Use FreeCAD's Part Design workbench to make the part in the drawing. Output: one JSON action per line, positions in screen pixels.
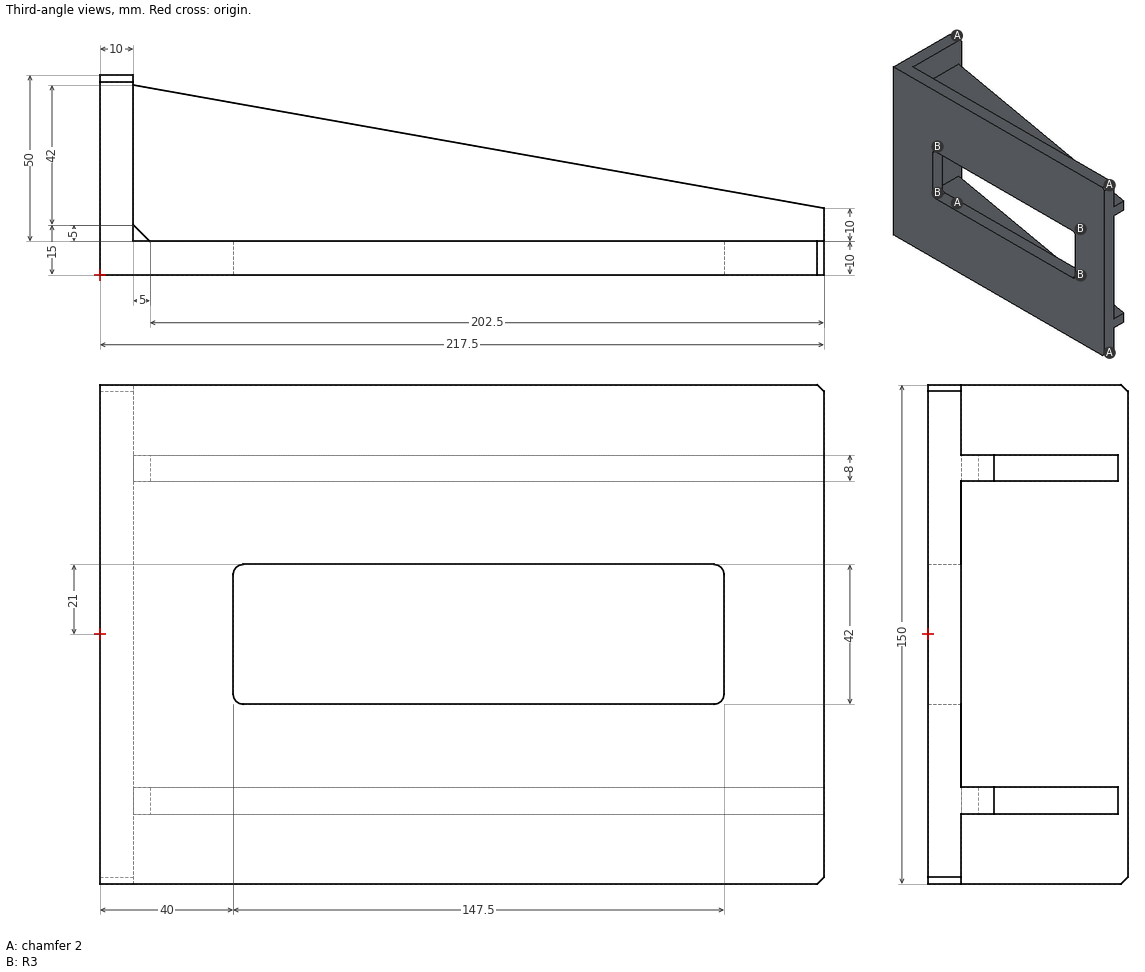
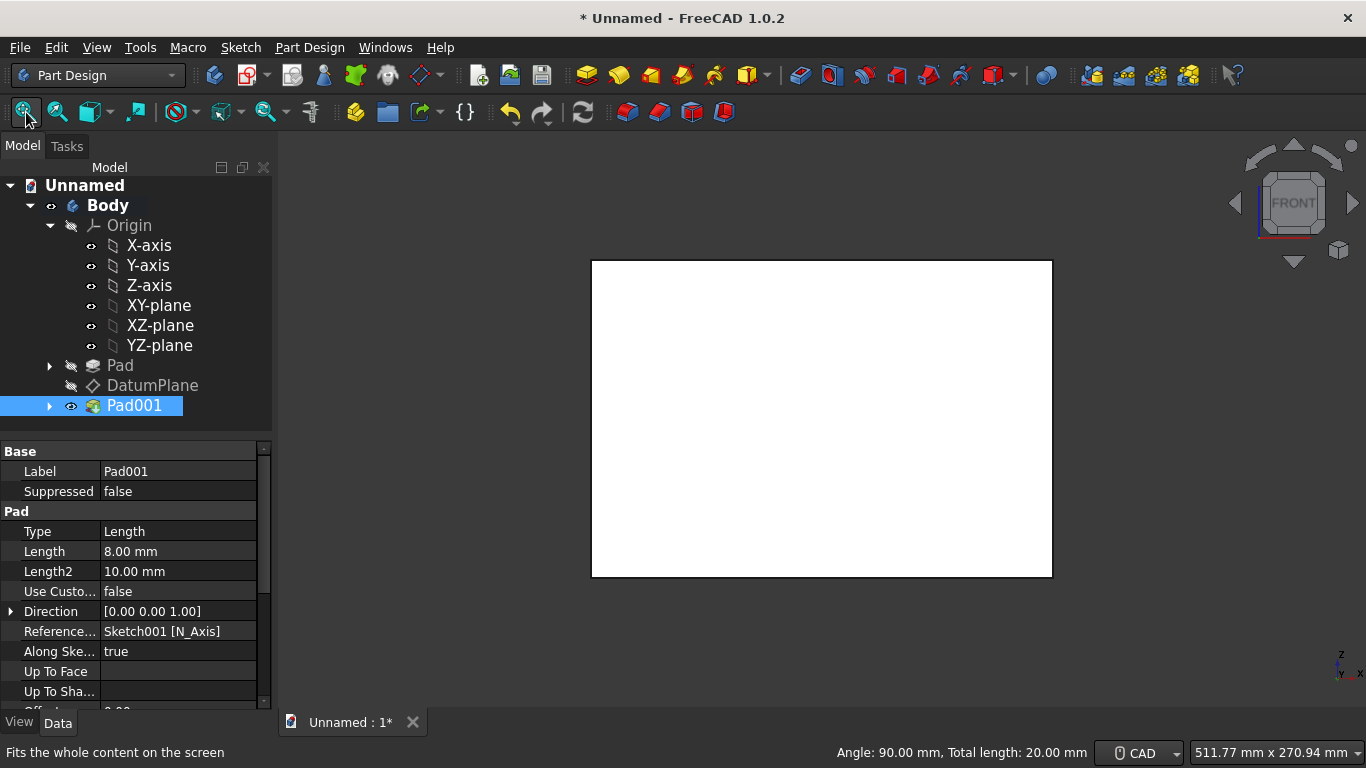
{"action": "scroll", "coordinate": [601, 577], "scroll_direction": "up", "scroll_amount": 4}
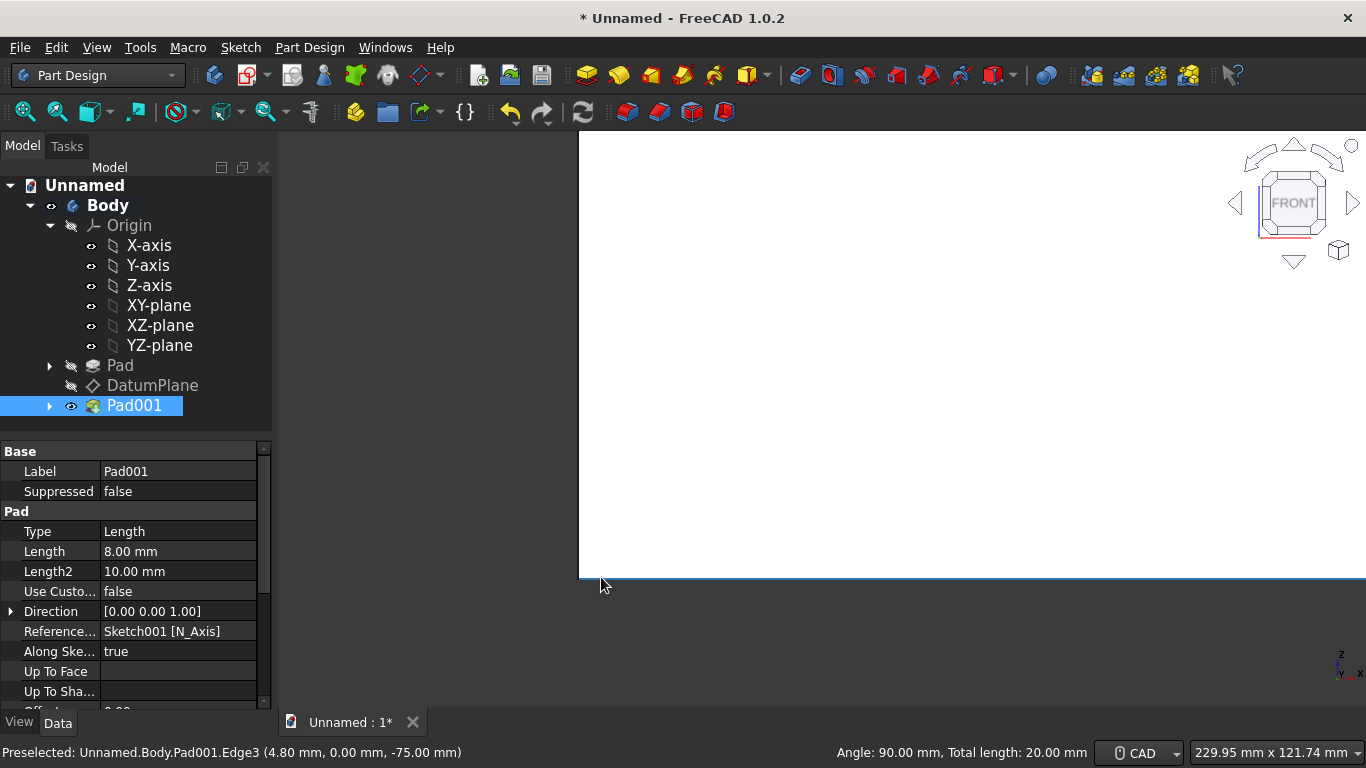
{"action": "left_click", "coordinate": [26, 112]}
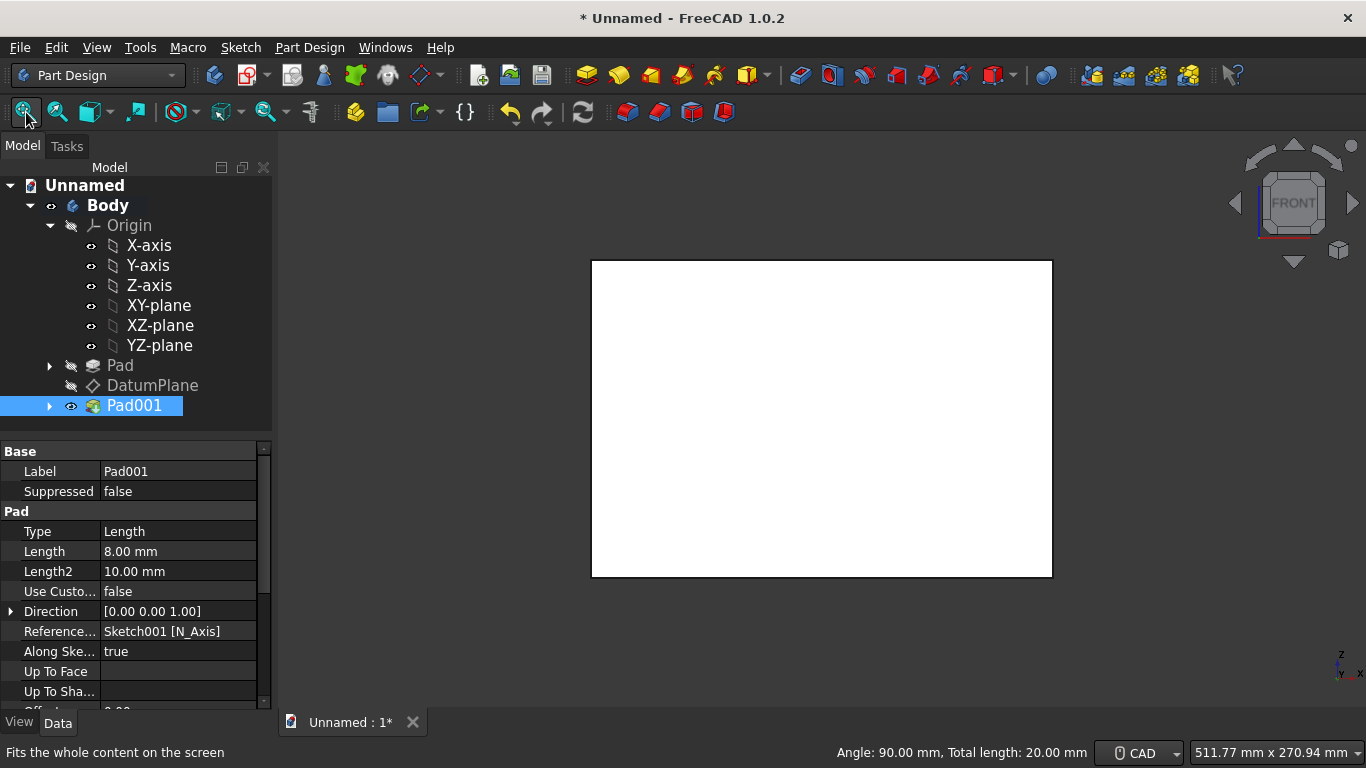
{"action": "key", "text": "3"}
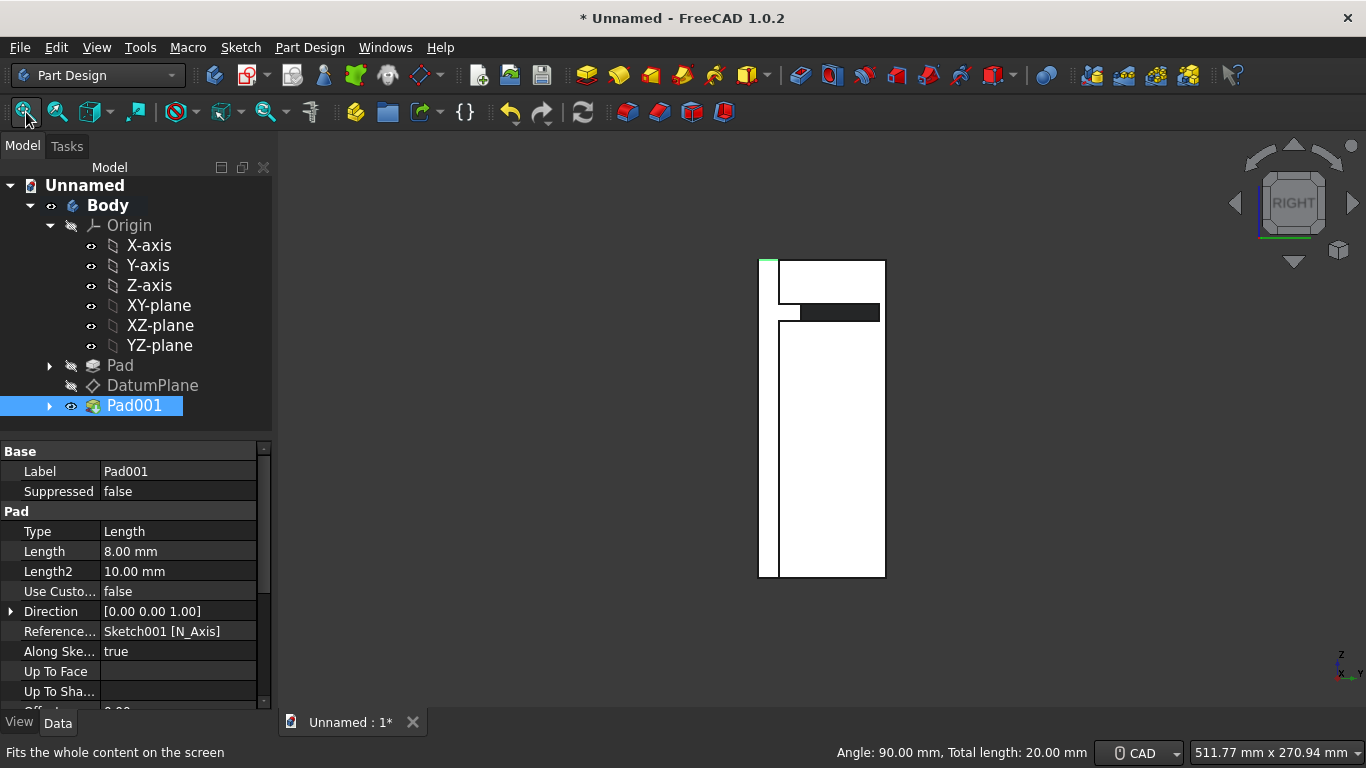
{"action": "left_click", "coordinate": [769, 577], "text": "ctrl"}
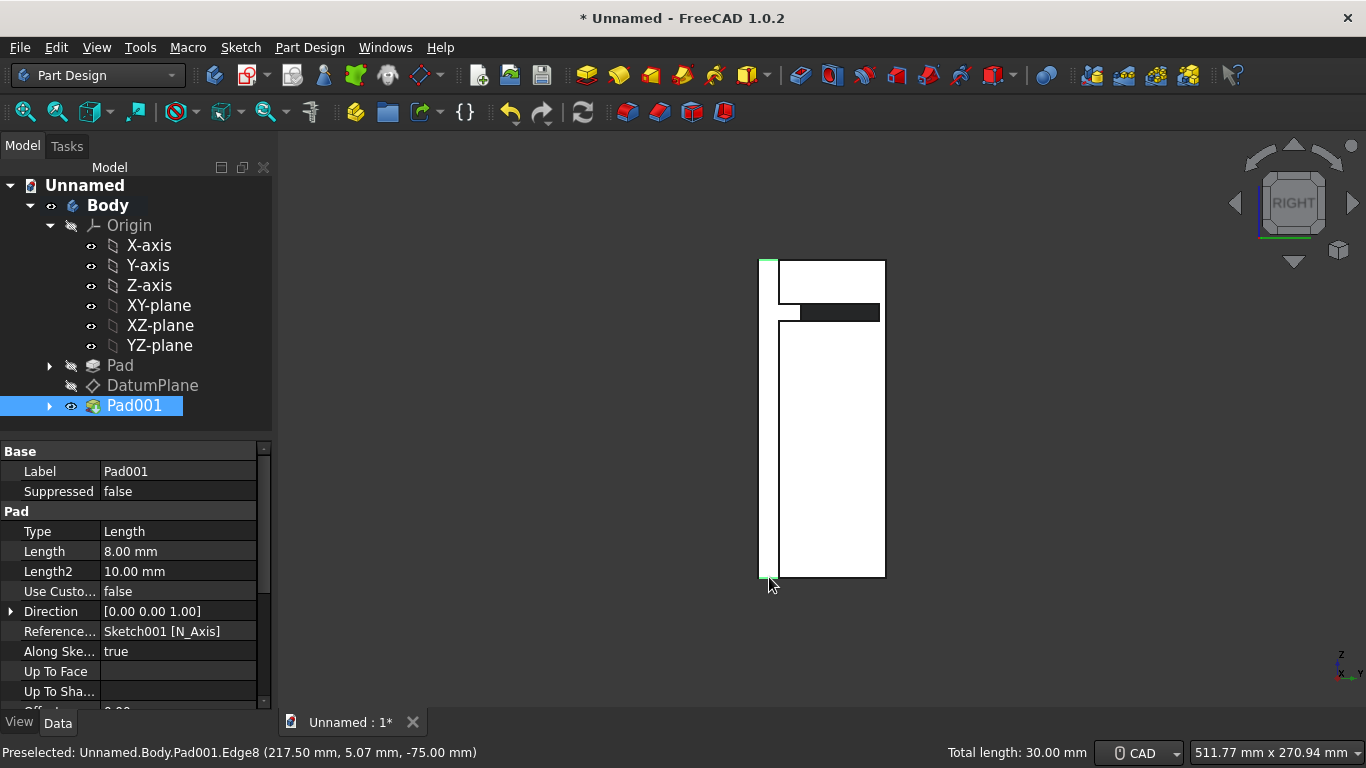
{"action": "scroll", "coordinate": [886, 577], "scroll_direction": "up", "scroll_amount": 4}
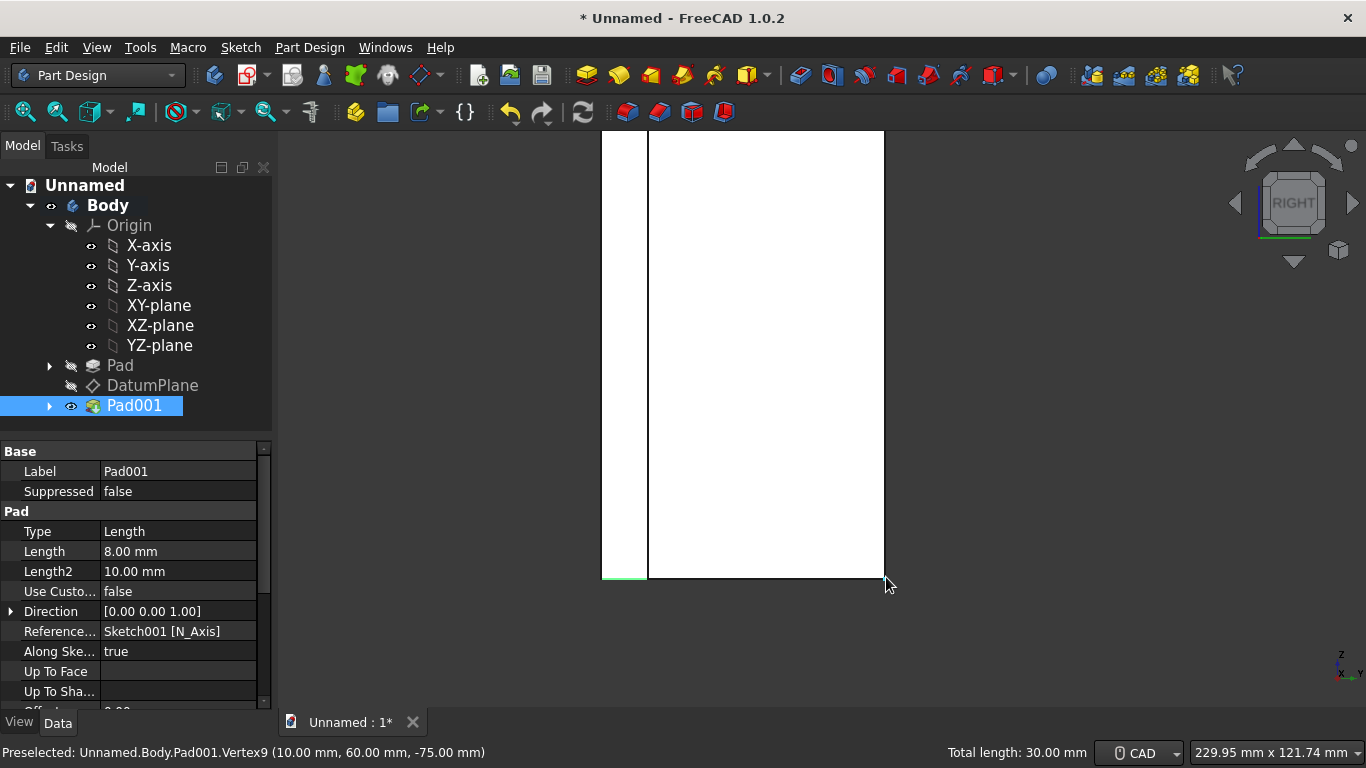
{"action": "left_click", "coordinate": [26, 112]}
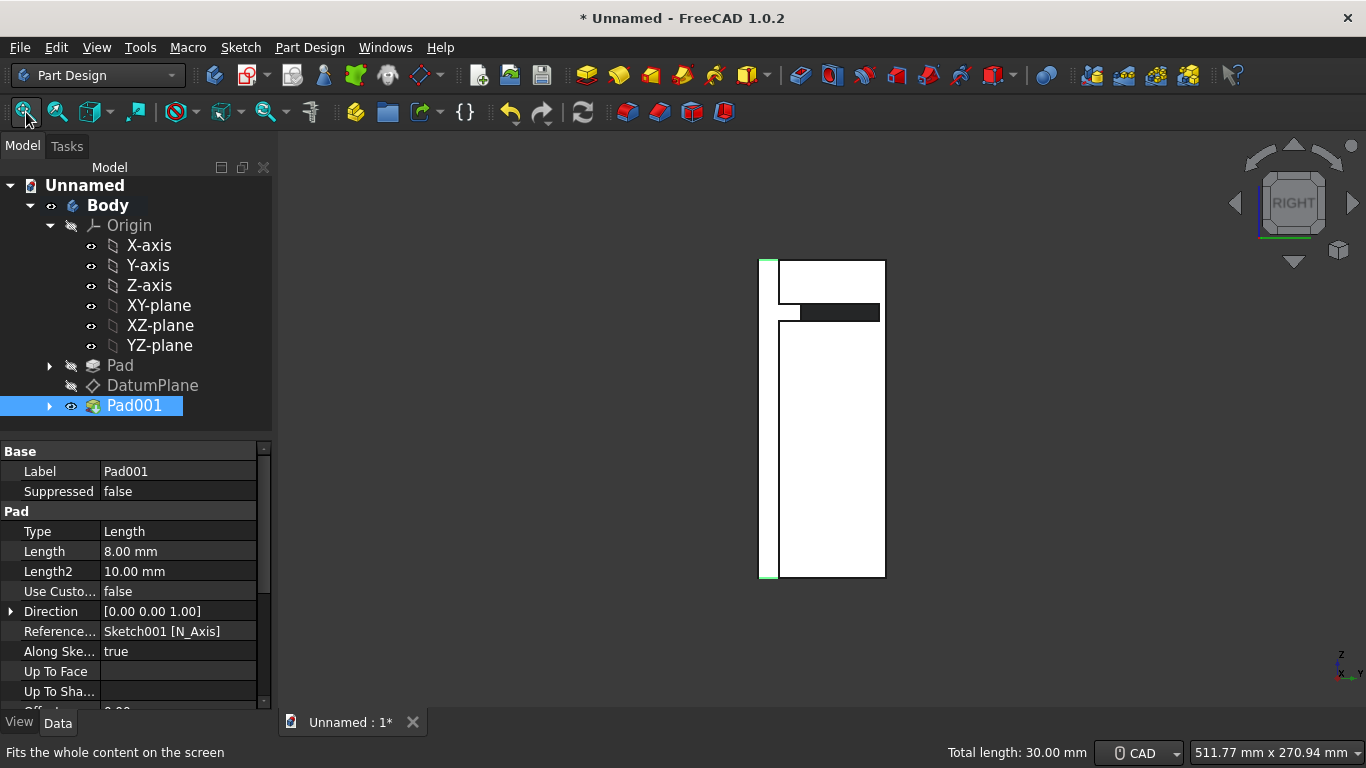
{"action": "key", "text": "5"}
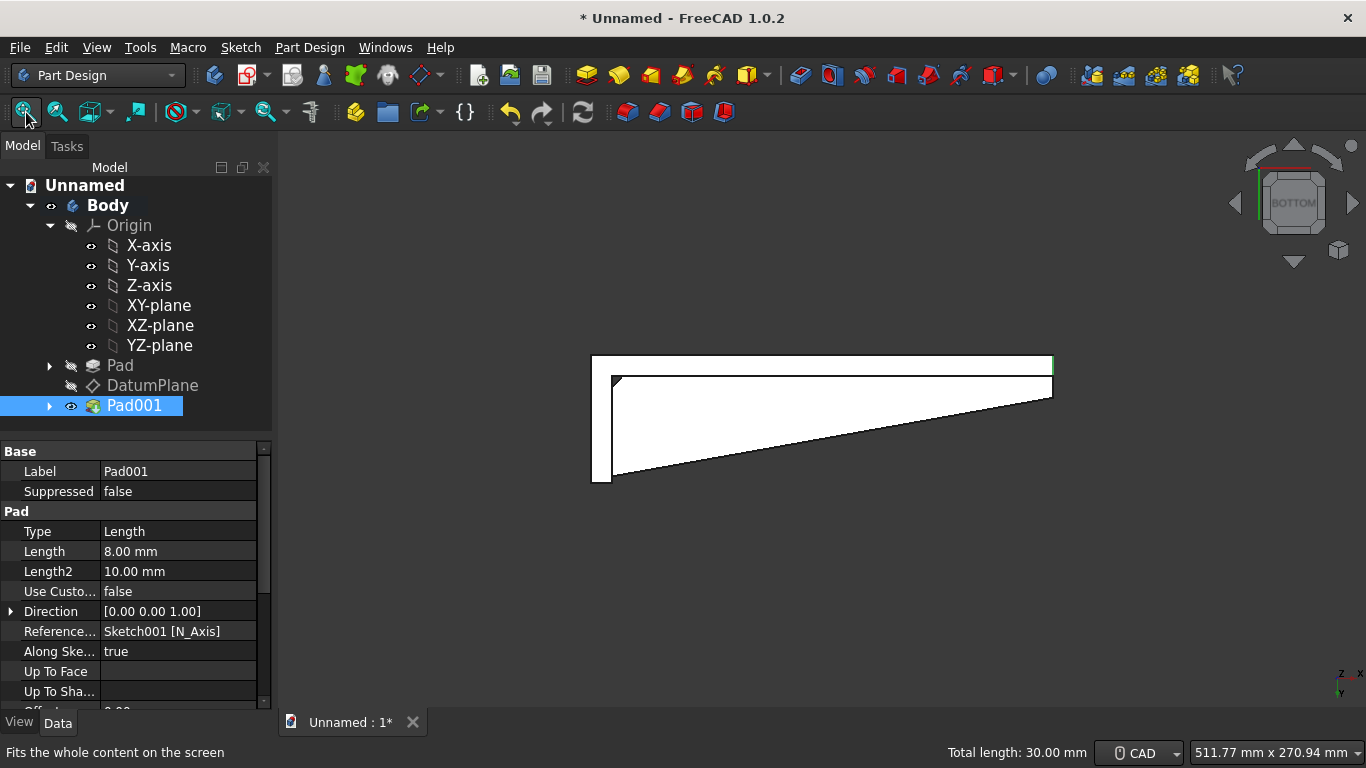
{"action": "left_click", "coordinate": [26, 112]}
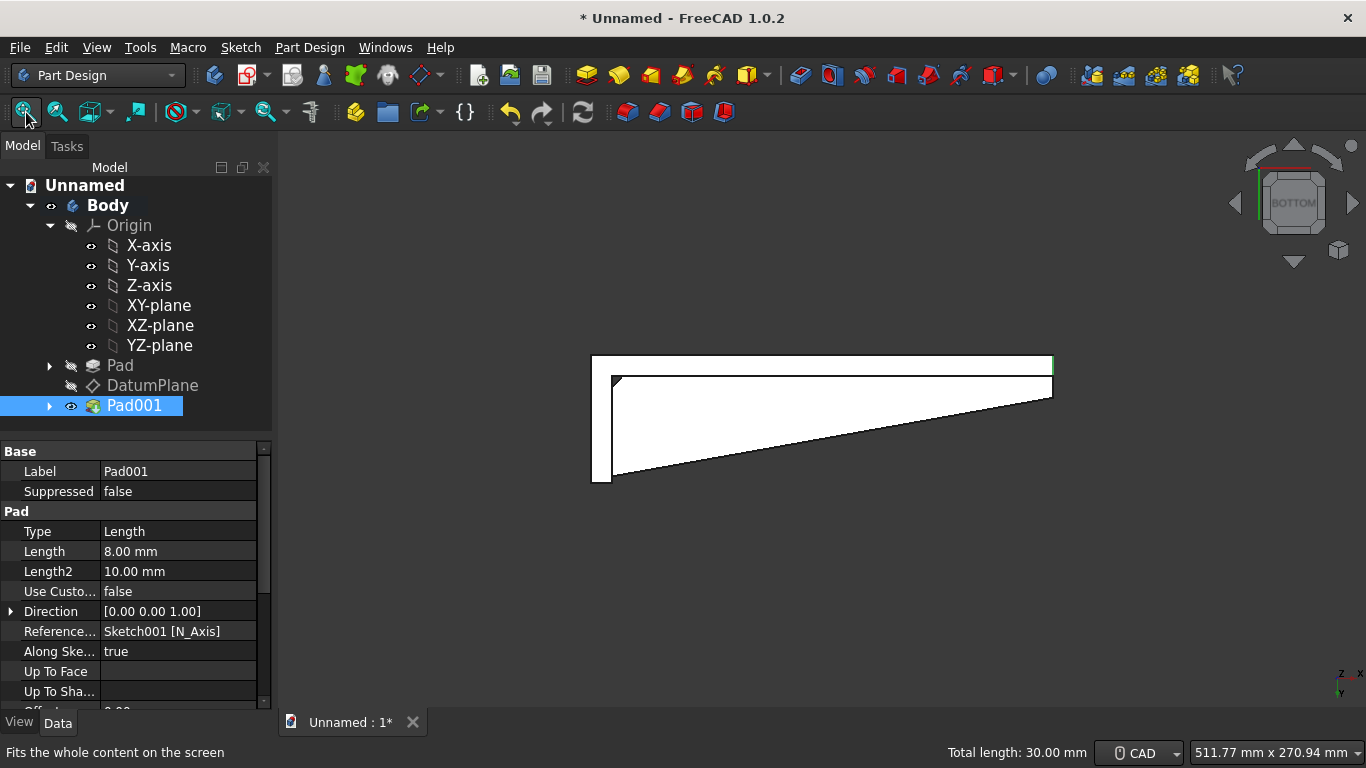
{"action": "left_click", "coordinate": [601, 482], "text": "ctrl"}